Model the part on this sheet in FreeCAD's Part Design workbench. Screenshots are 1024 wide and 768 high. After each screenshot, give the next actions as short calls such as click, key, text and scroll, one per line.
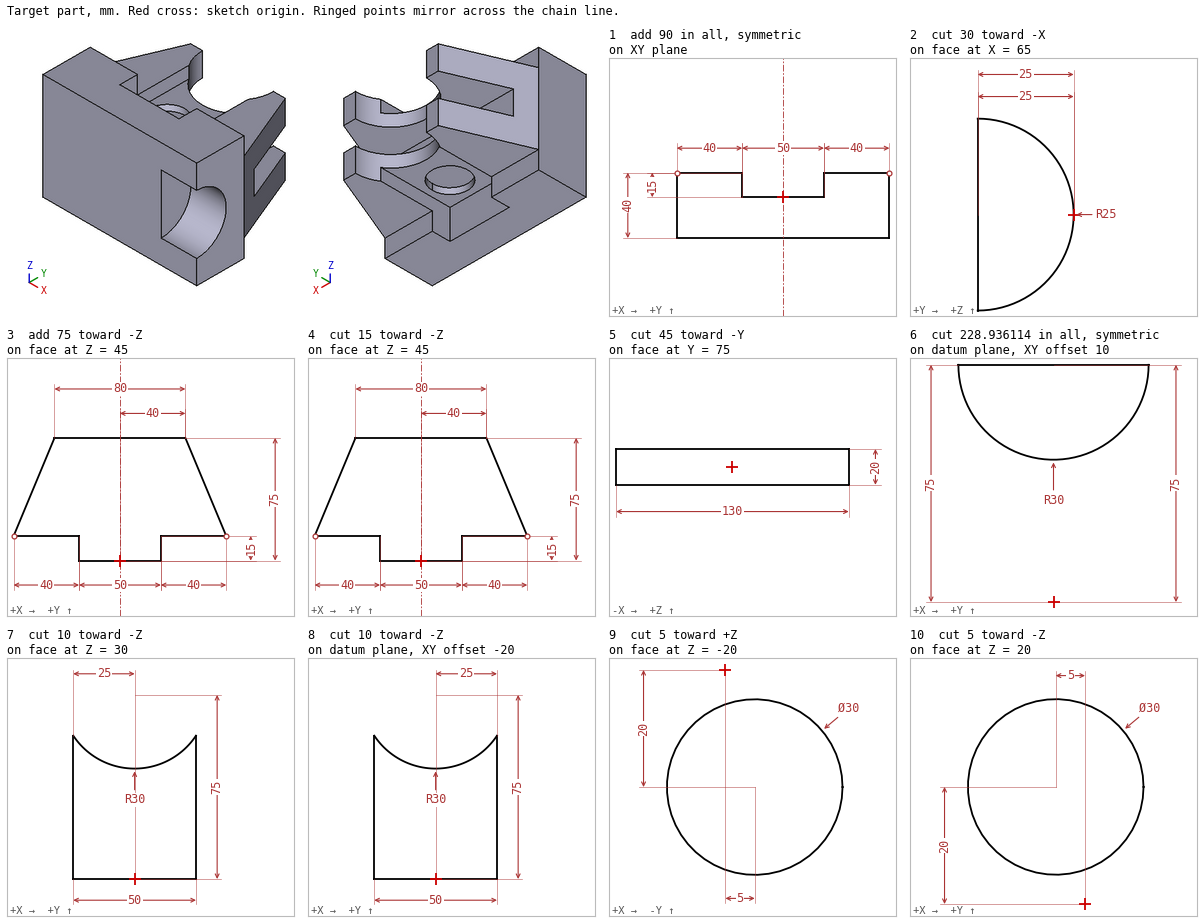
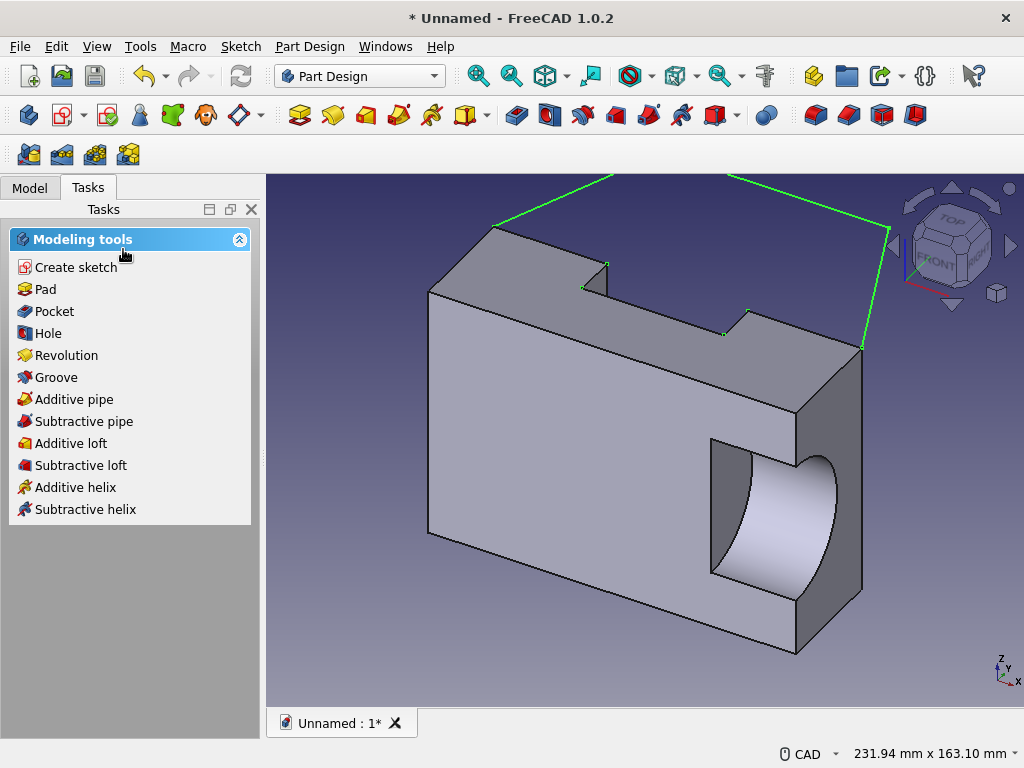
click(300, 116)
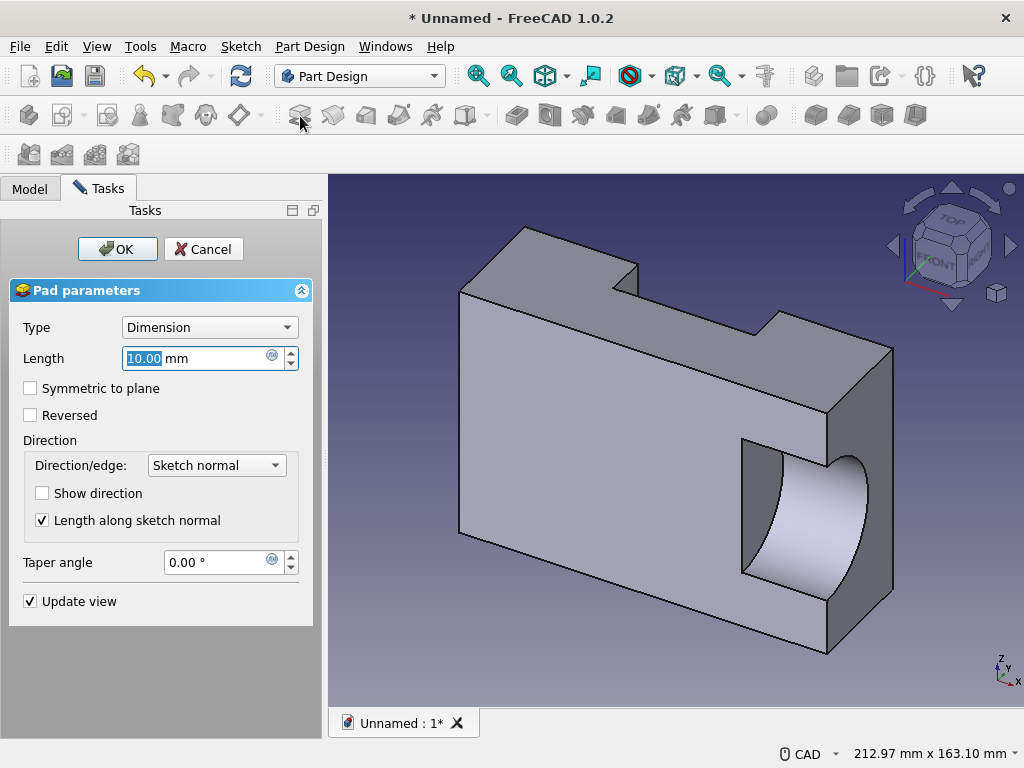
text(75)
key(Tab)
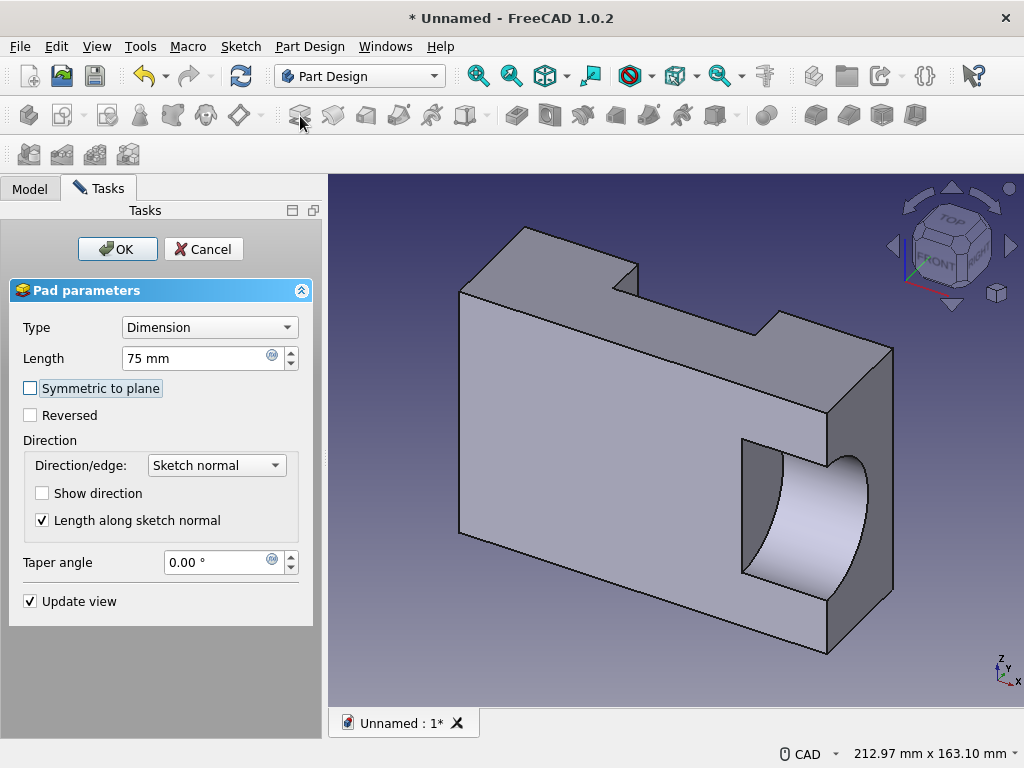
click(31, 415)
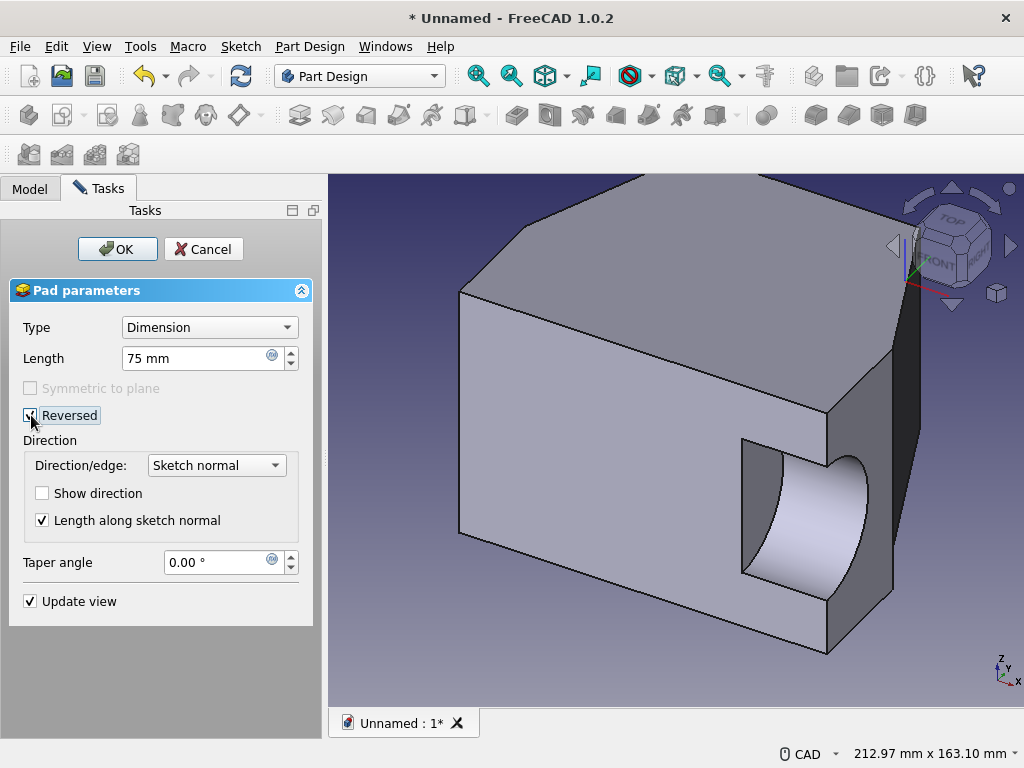
click(118, 249)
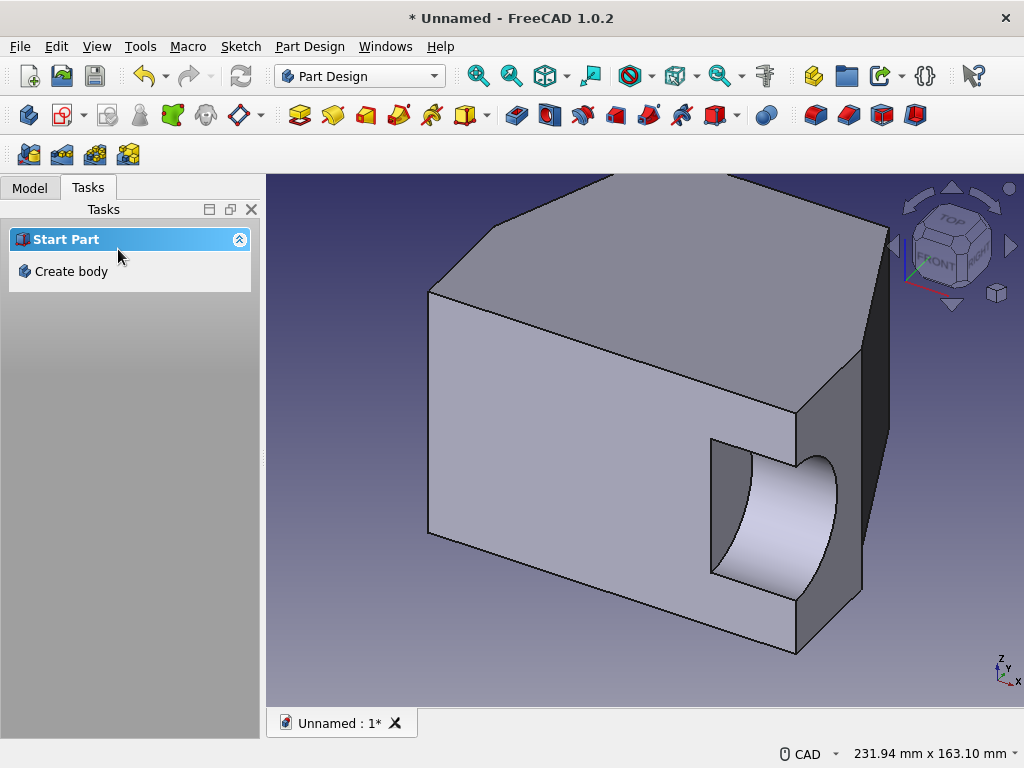
key(v)
key(f)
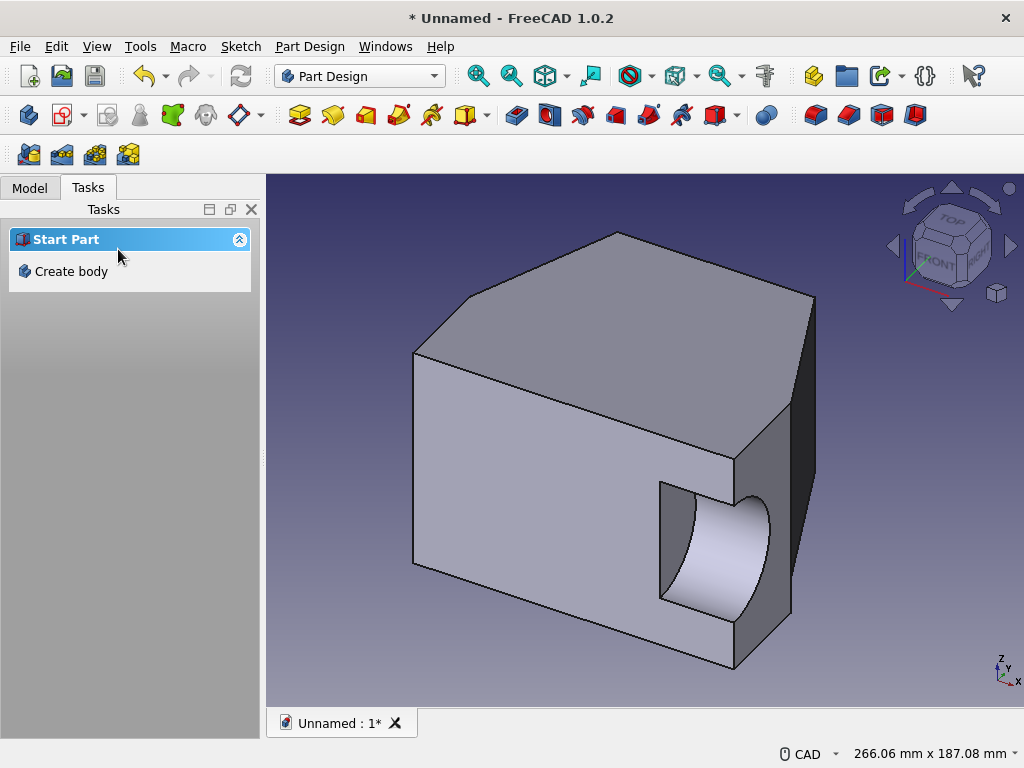
click(645, 334)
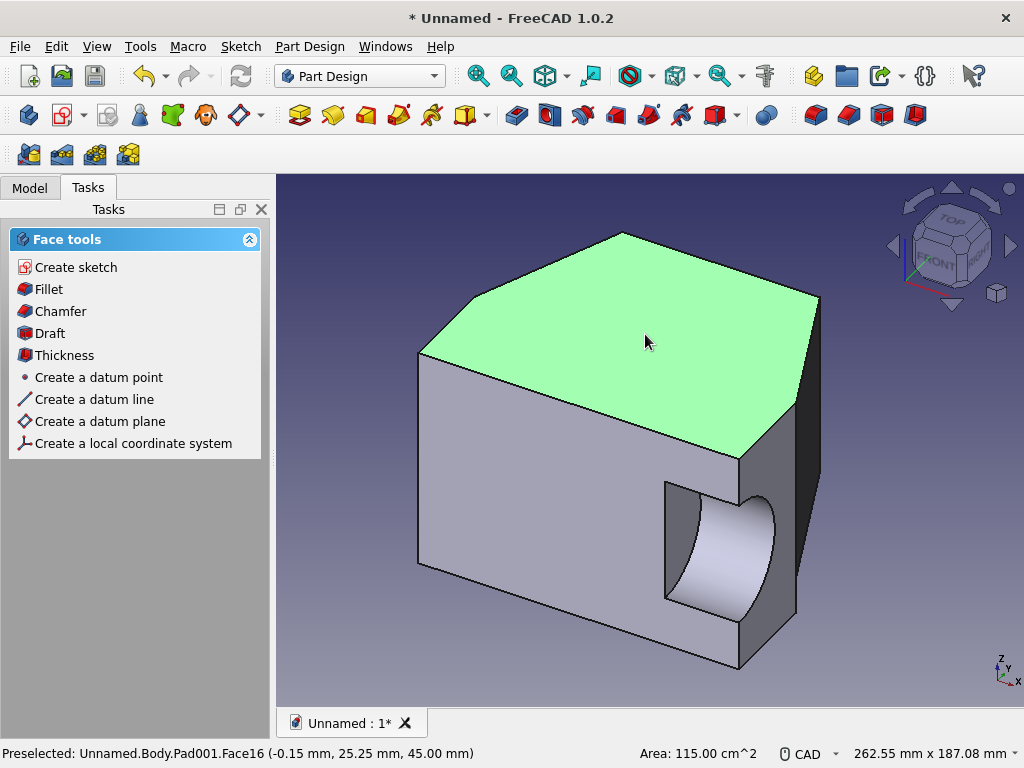
click(62, 116)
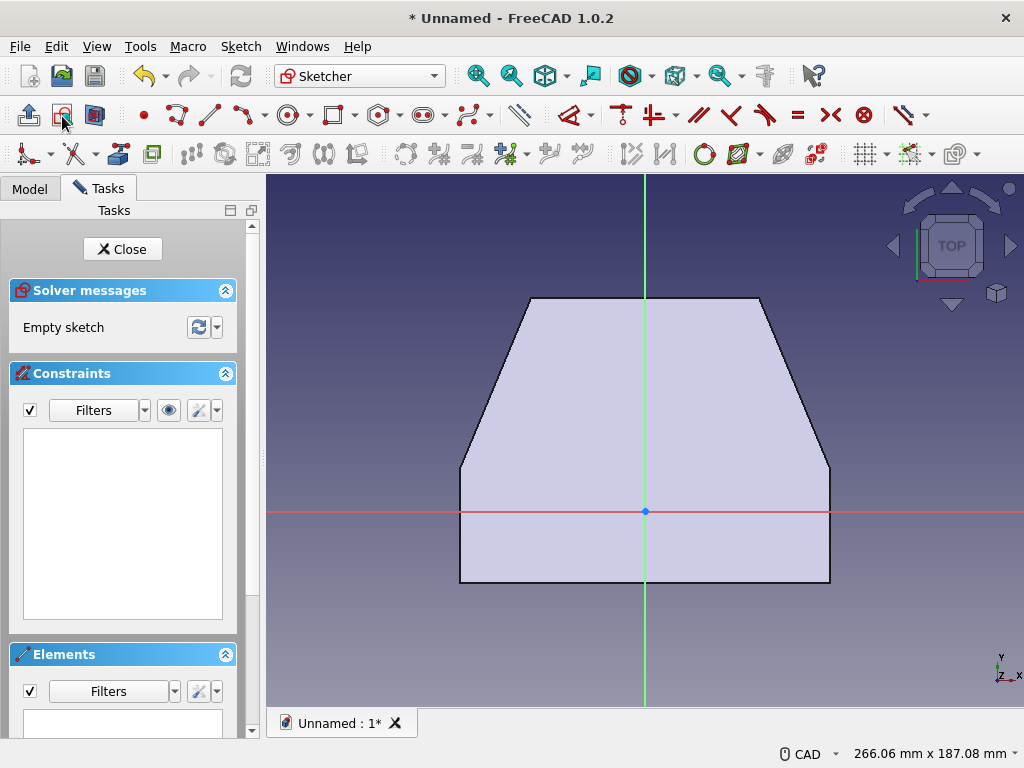
key(g)
key(m)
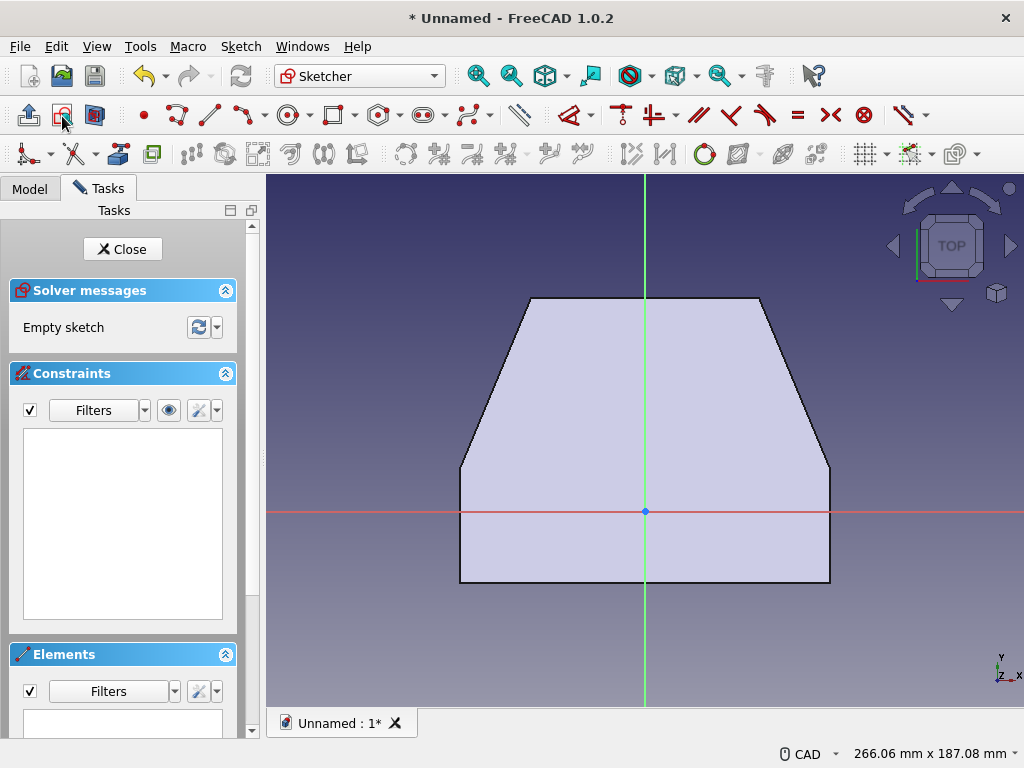
click(574, 512)
click(716, 503)
click(716, 469)
click(830, 469)
click(759, 298)
click(531, 298)
click(460, 469)
click(574, 469)
click(574, 512)
key(Escape)
key(Escape)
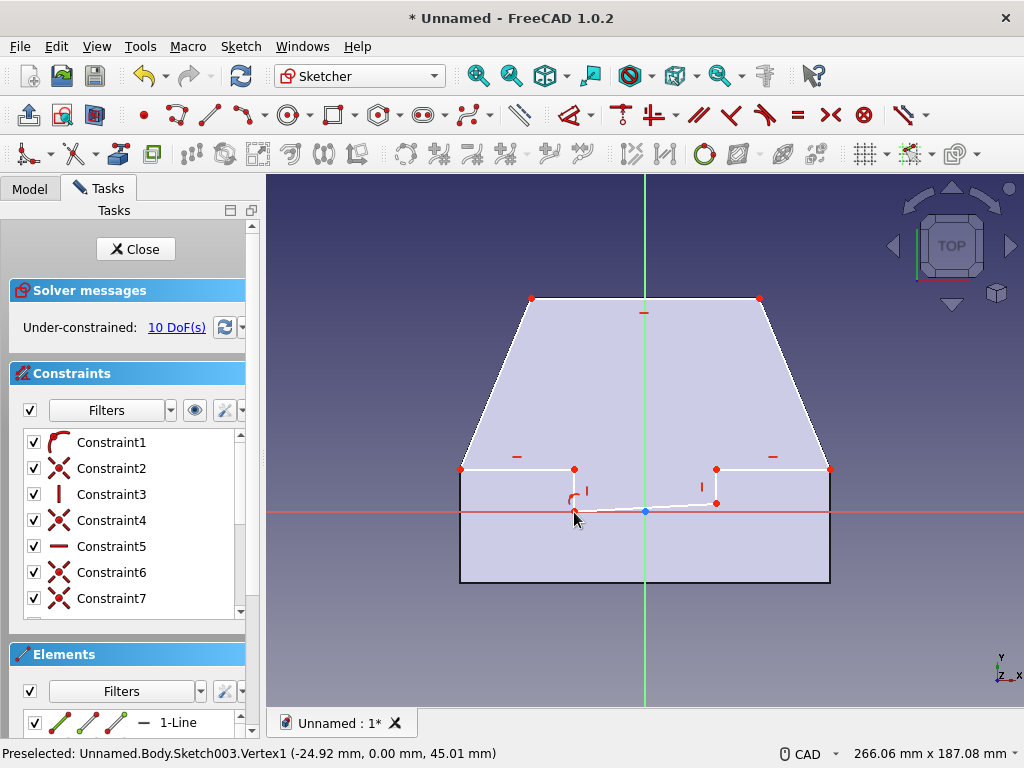
click(617, 509)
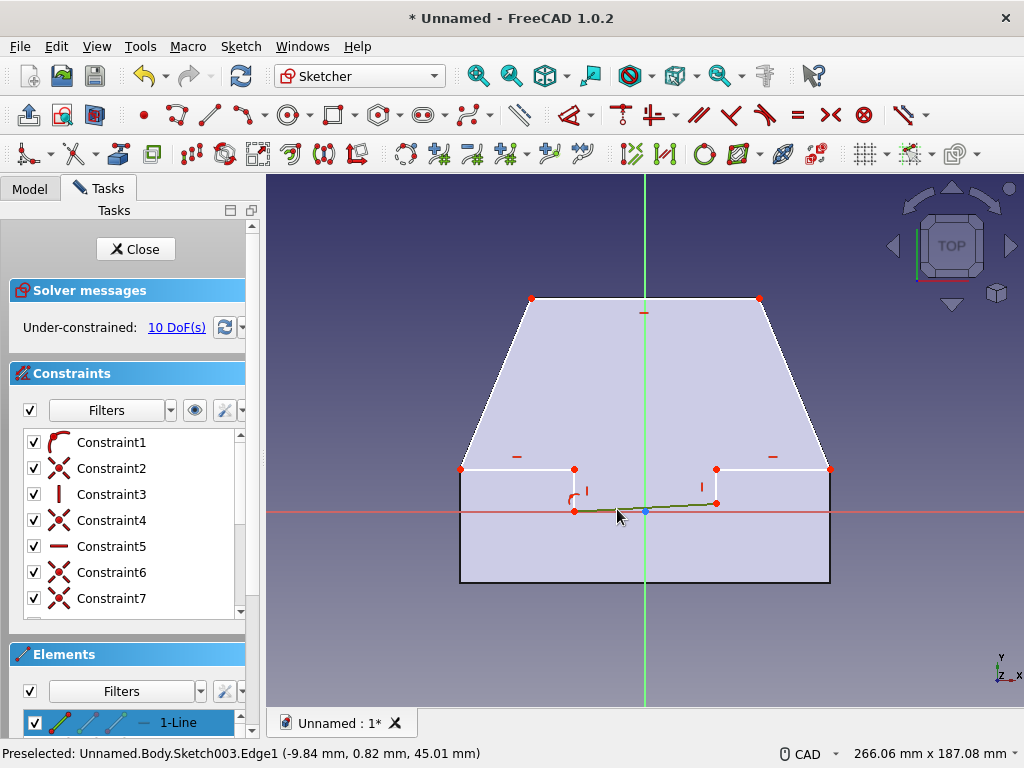
click(676, 116)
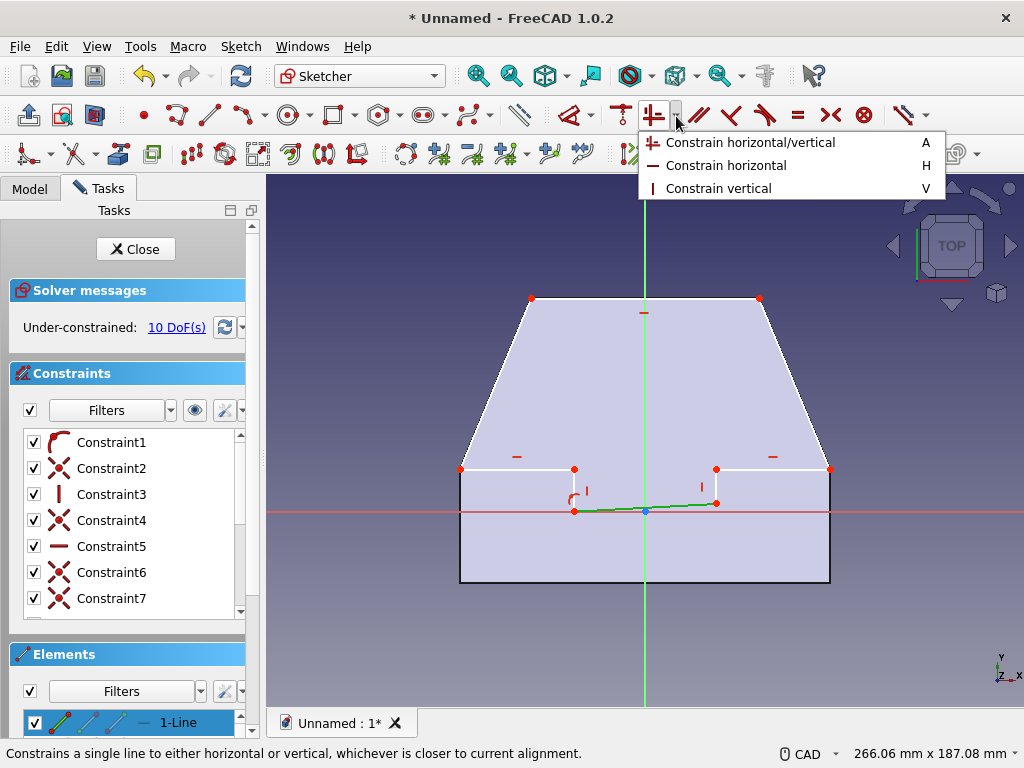
click(792, 166)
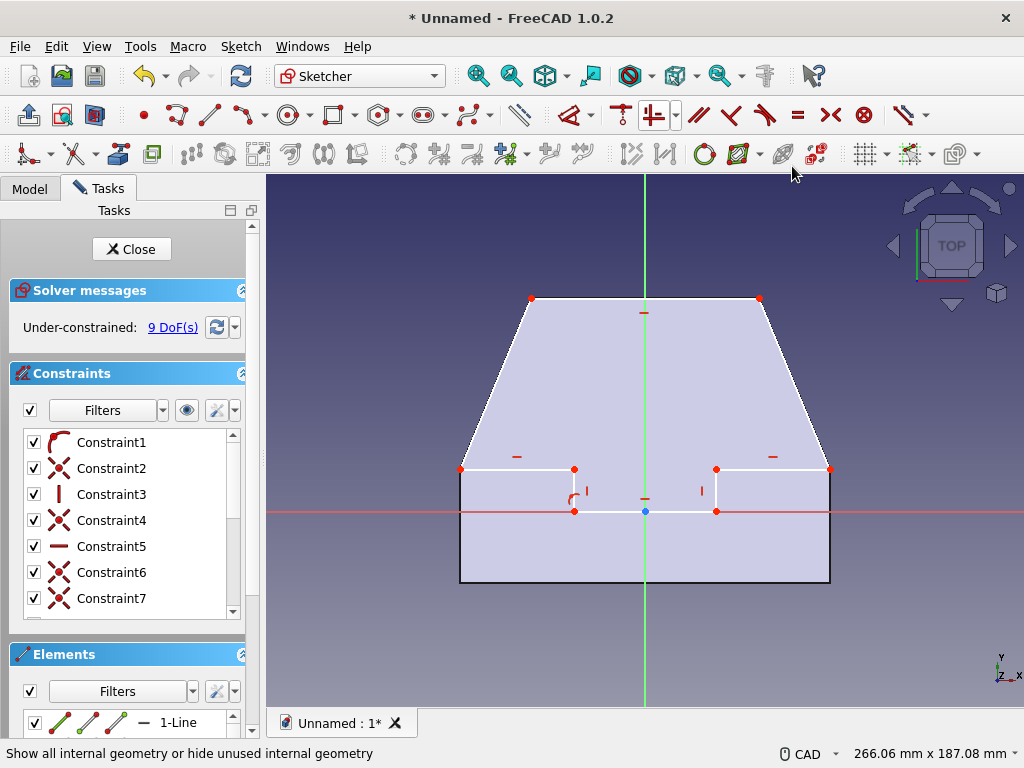
click(830, 470)